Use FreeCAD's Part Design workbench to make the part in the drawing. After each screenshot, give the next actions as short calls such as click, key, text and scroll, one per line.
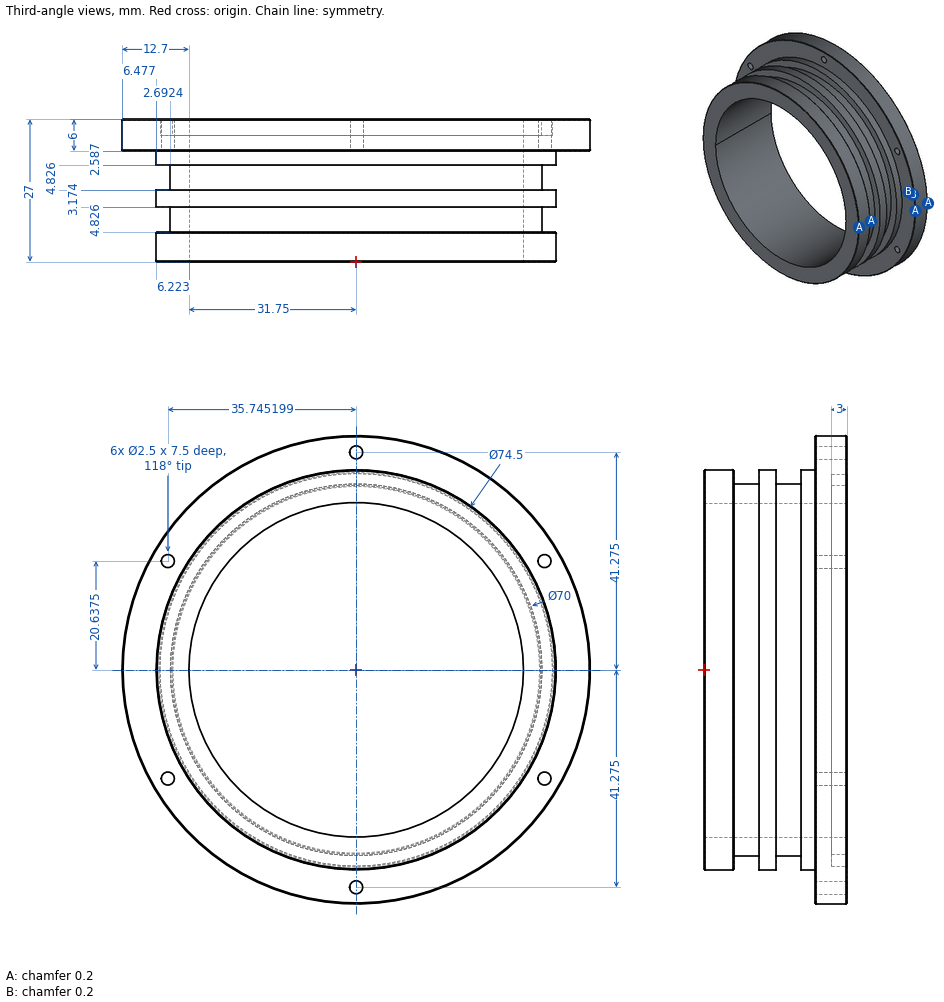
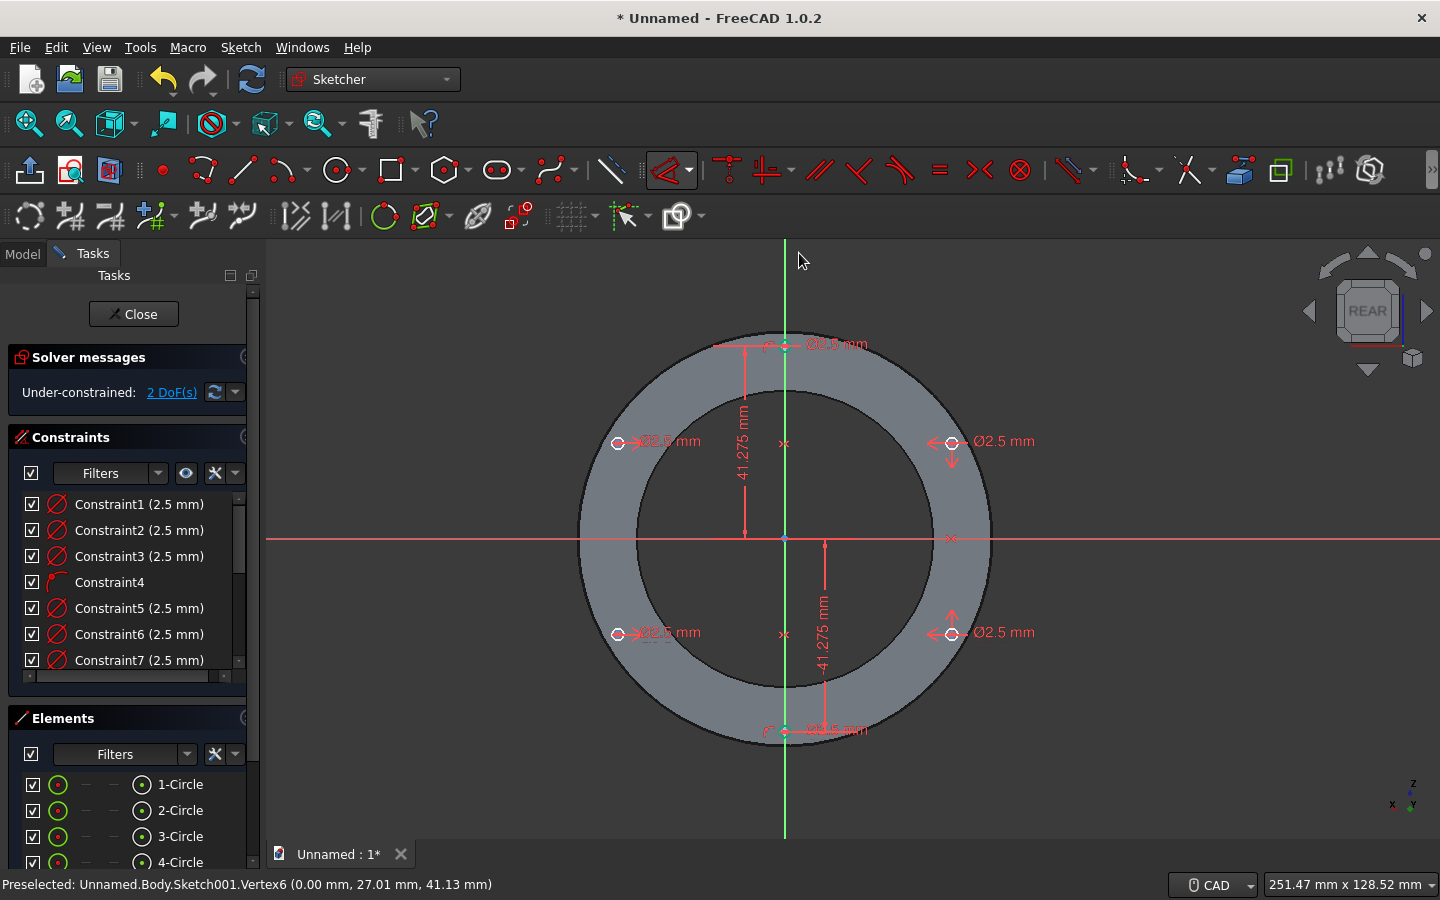
click(952, 443)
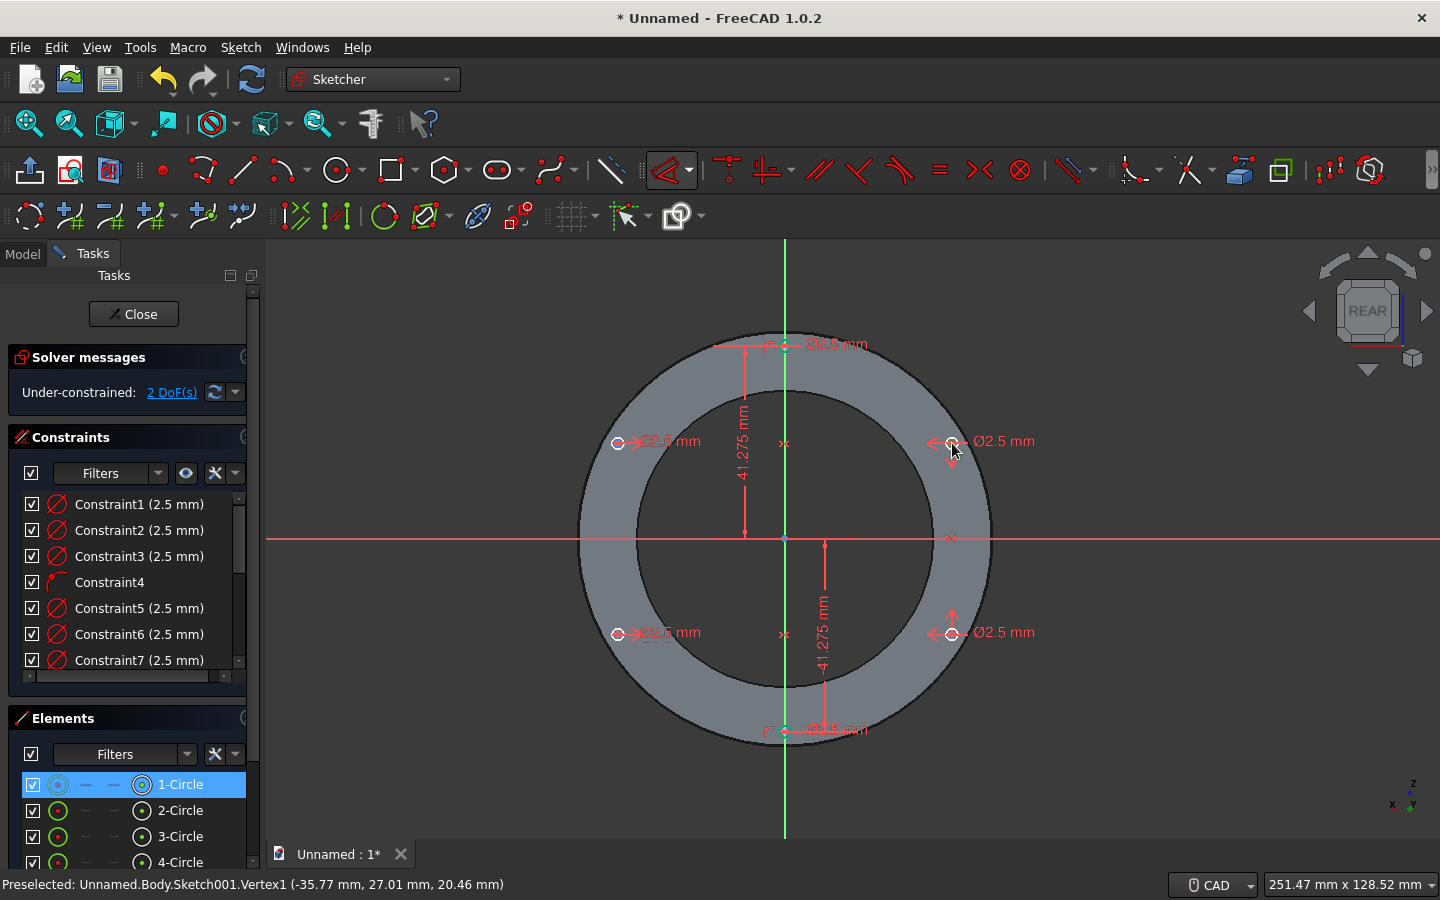
key(i)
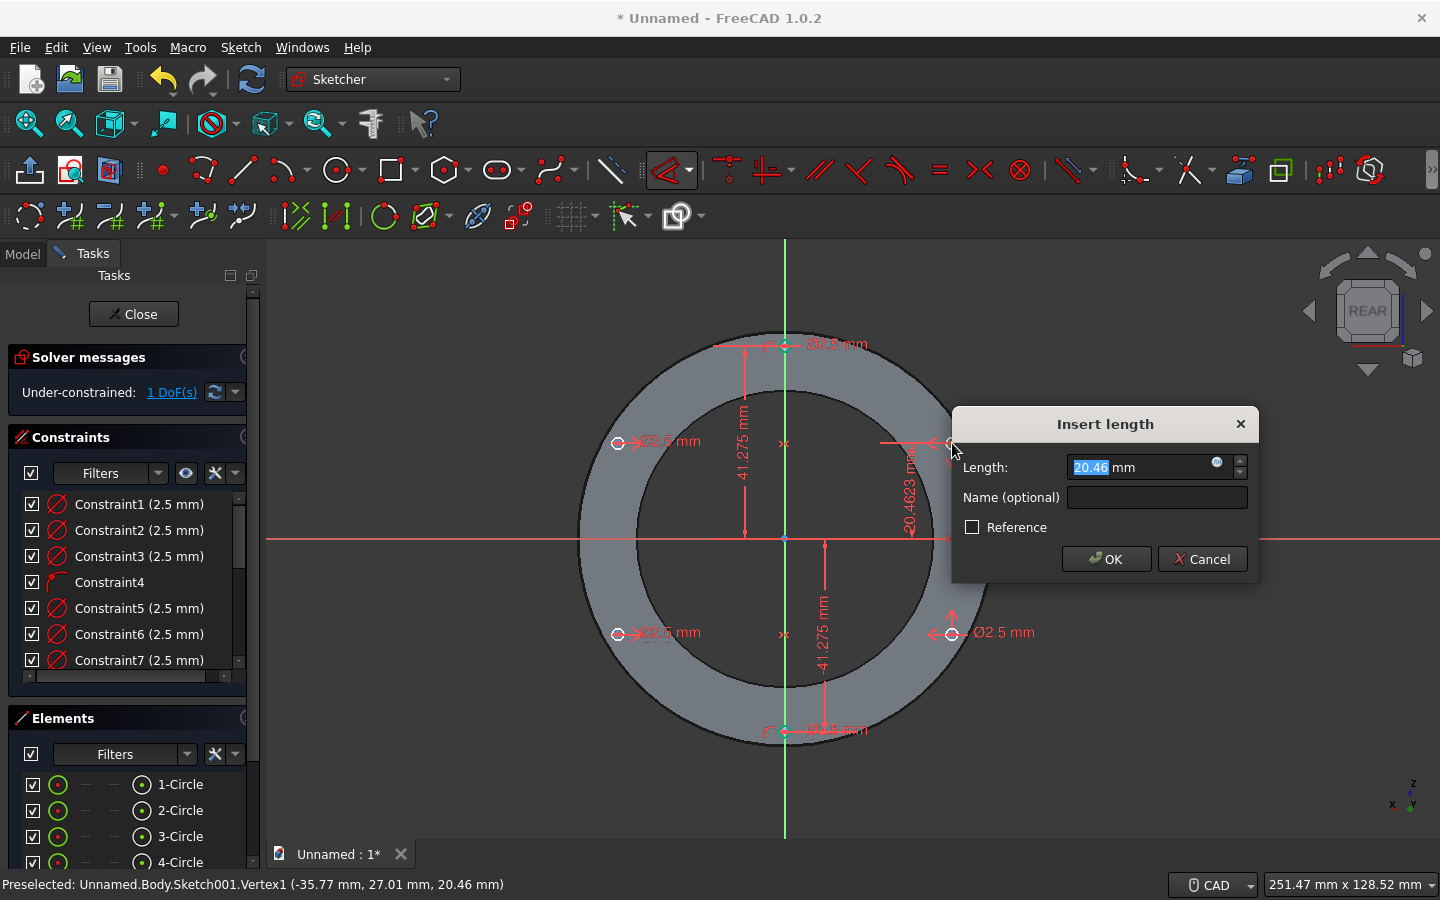
text(20.6375)
key(Return)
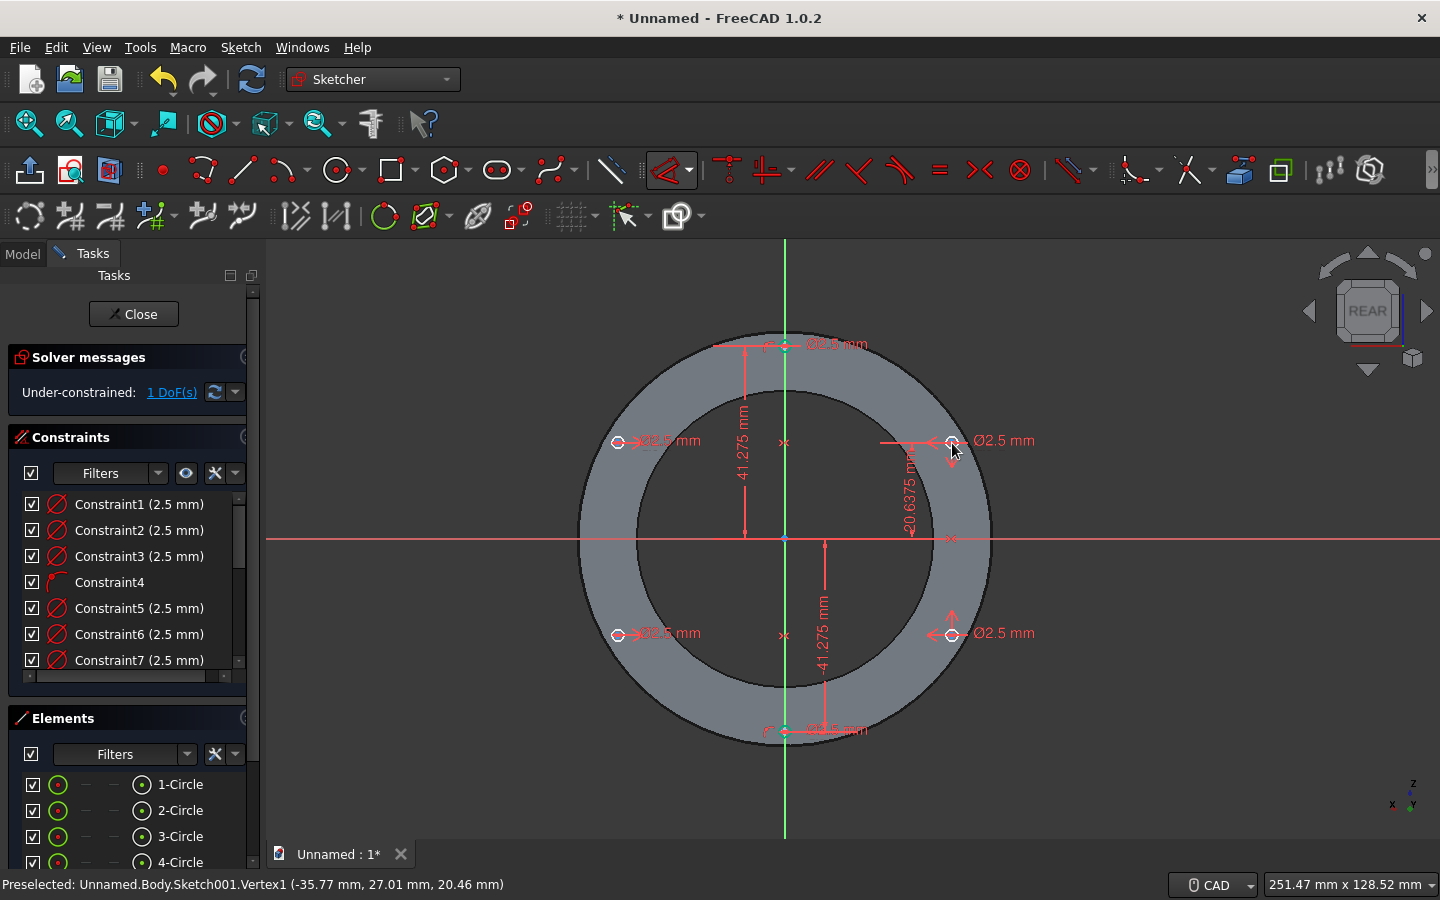
click(952, 443)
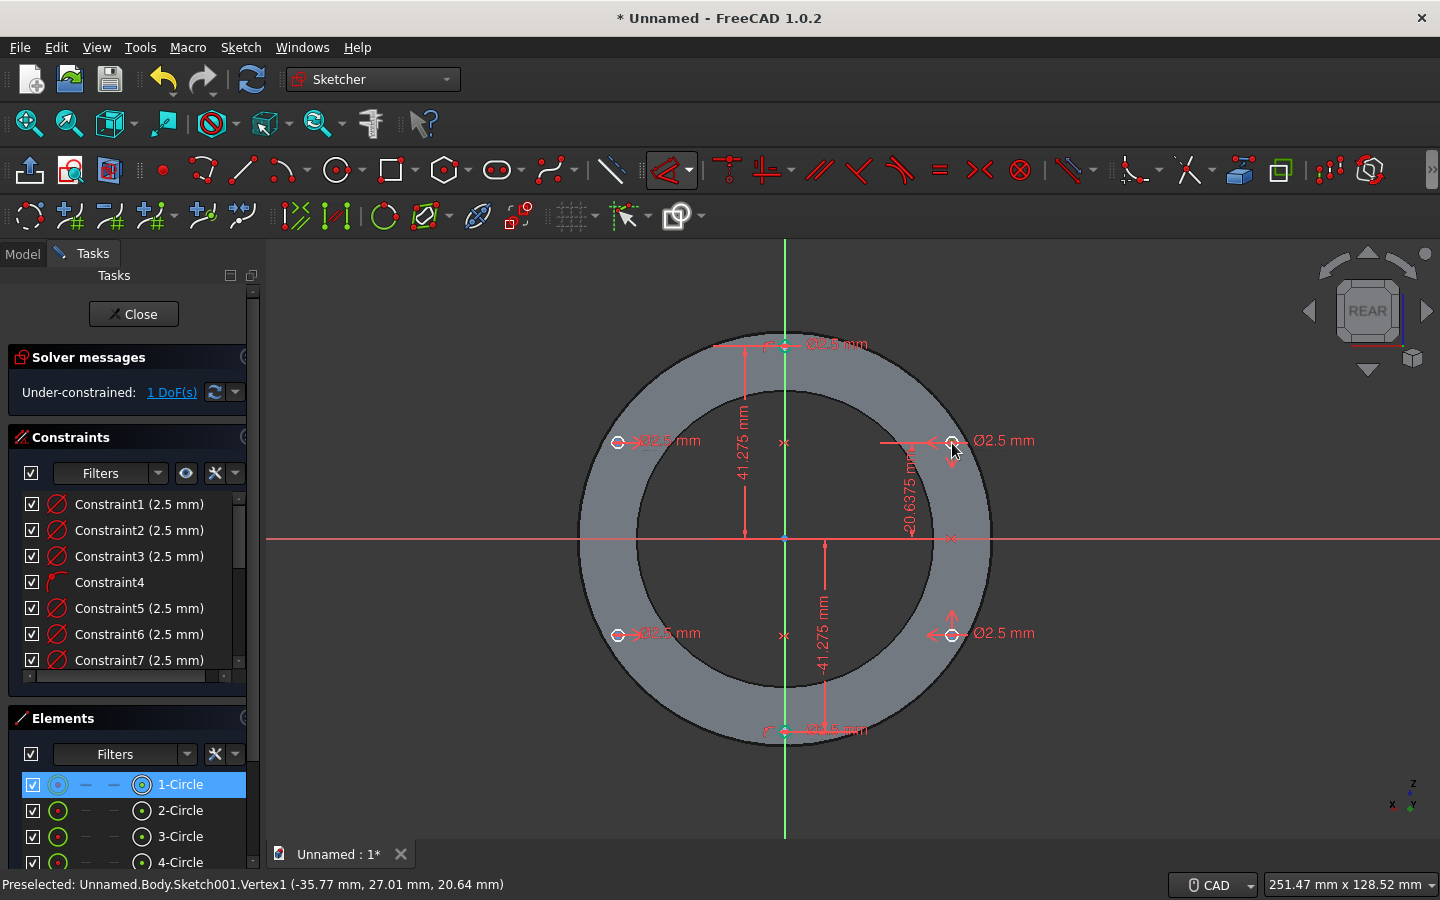
key(l)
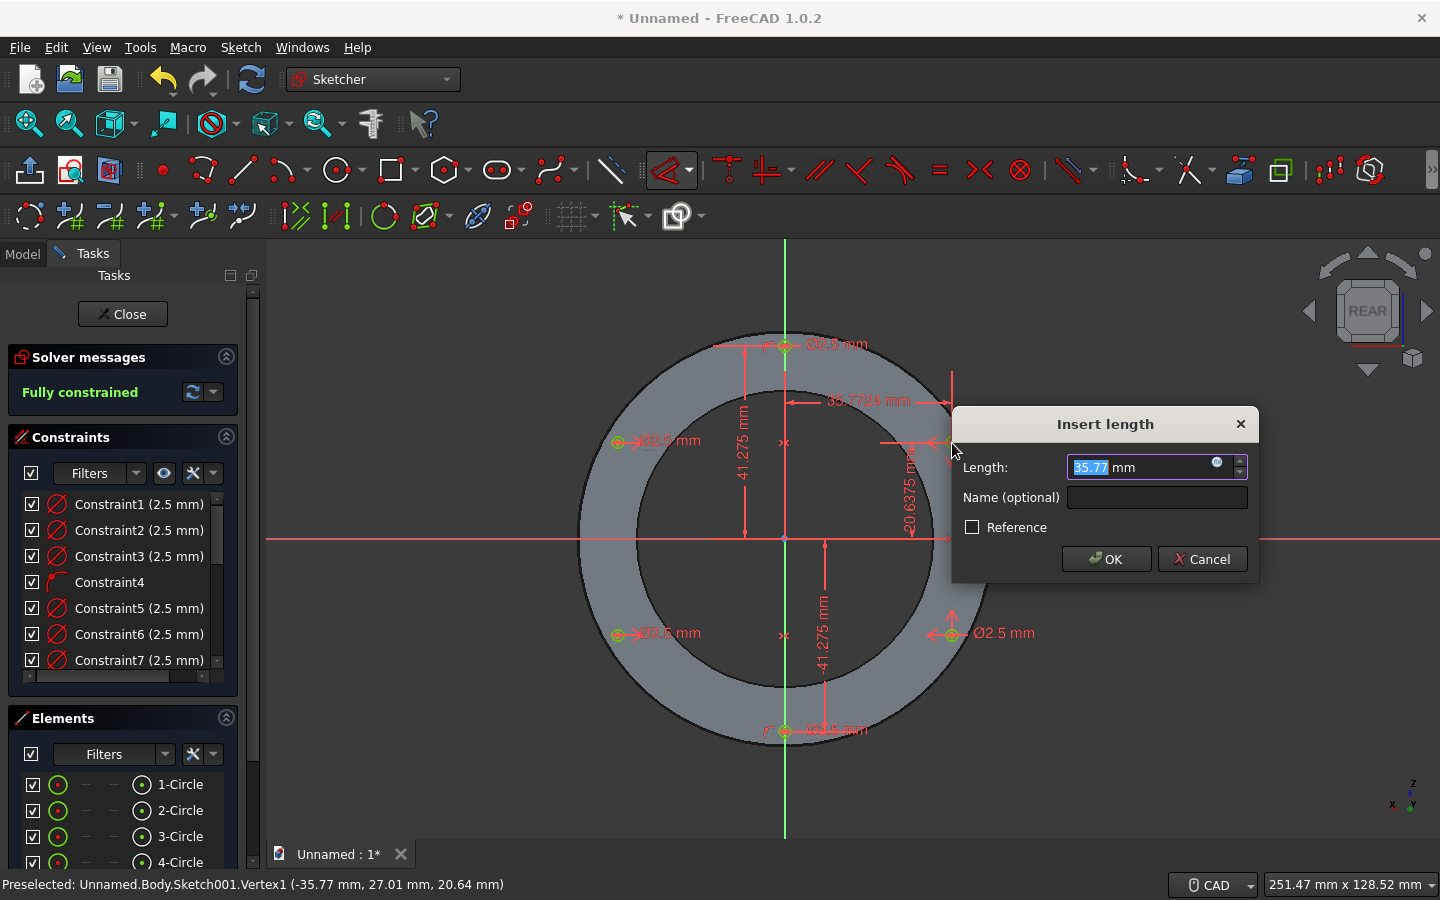
text(35.745199)
key(Return)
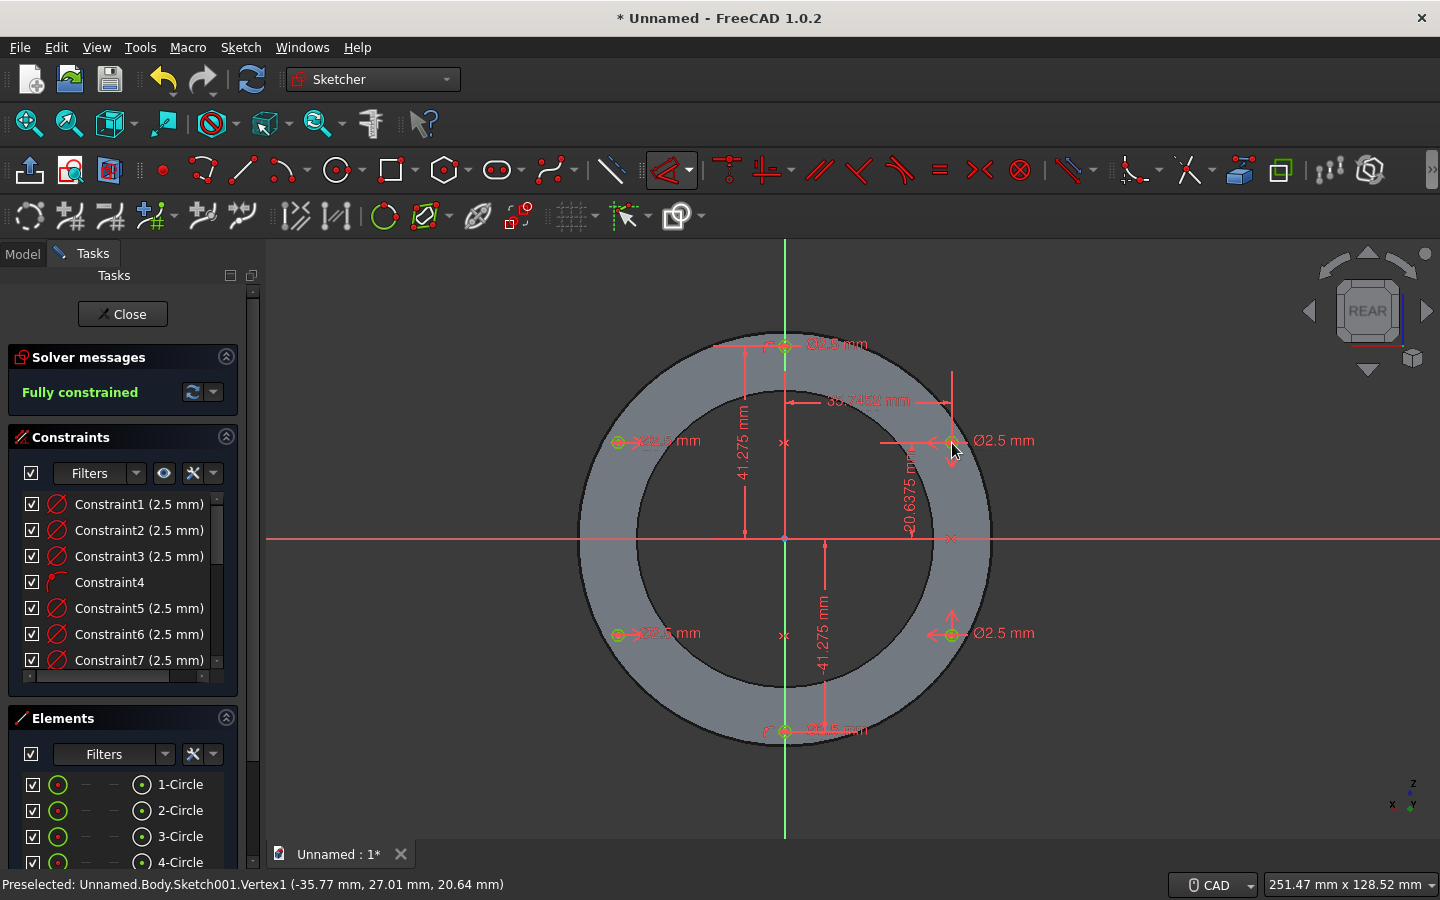
click(123, 314)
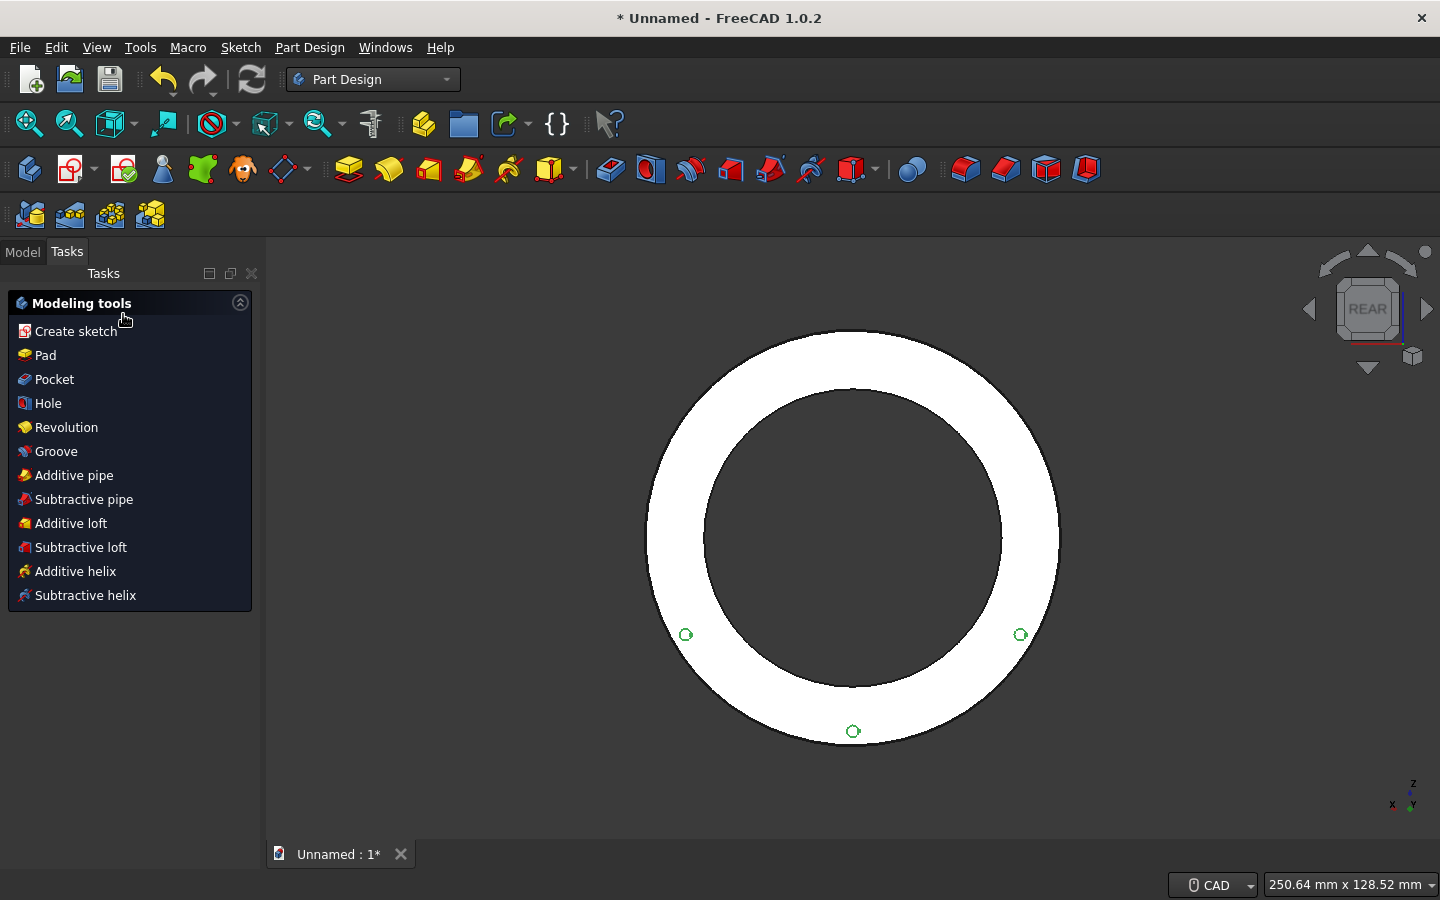
click(652, 170)